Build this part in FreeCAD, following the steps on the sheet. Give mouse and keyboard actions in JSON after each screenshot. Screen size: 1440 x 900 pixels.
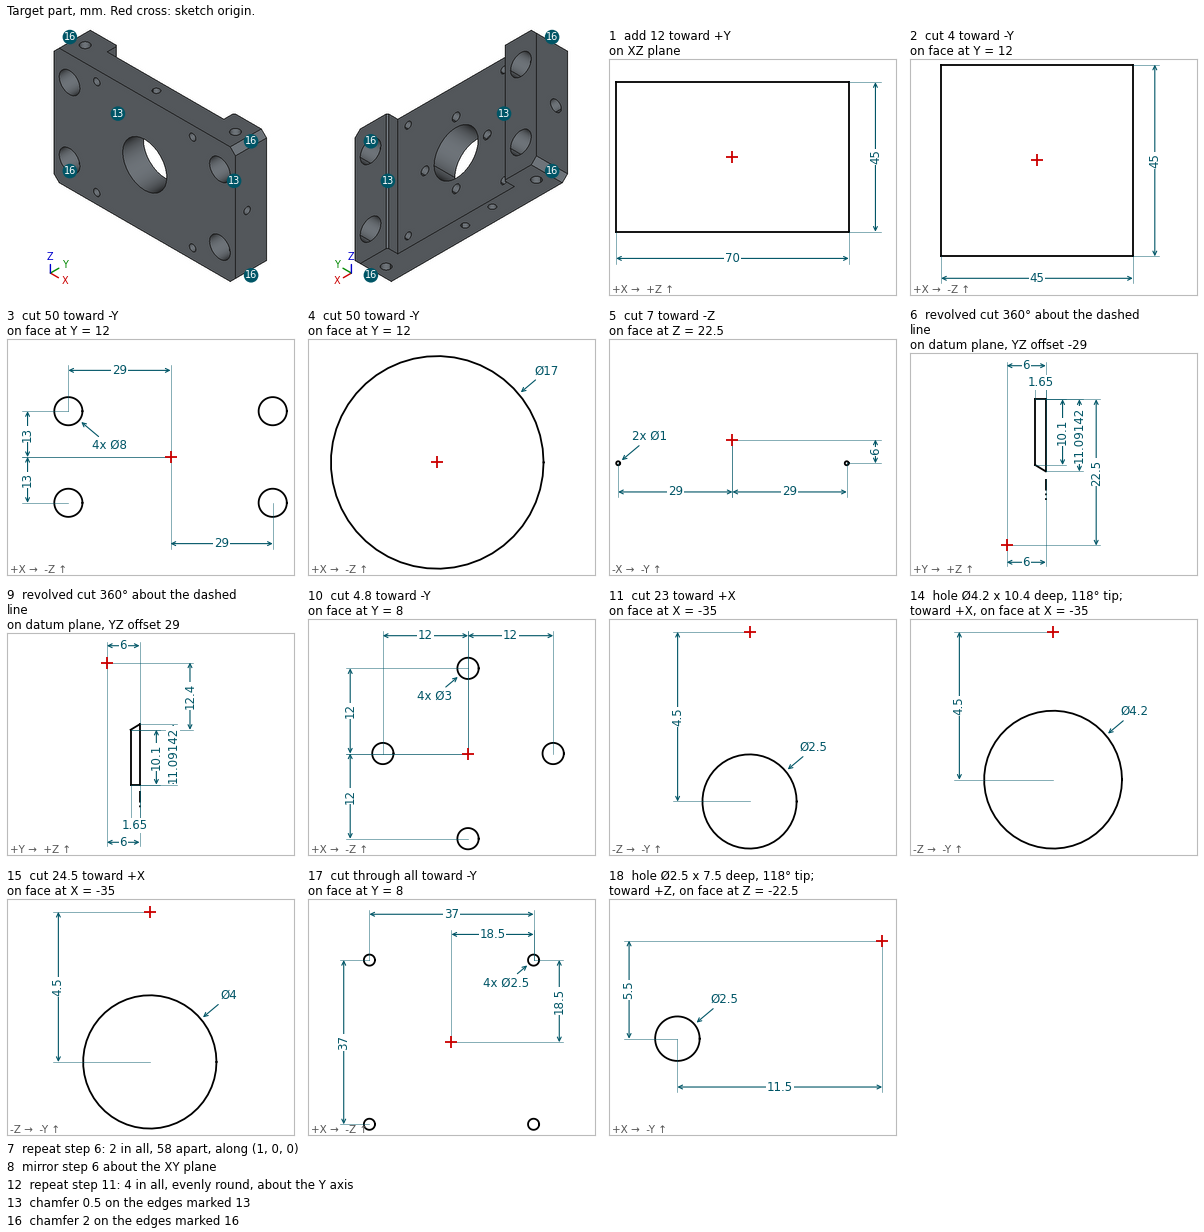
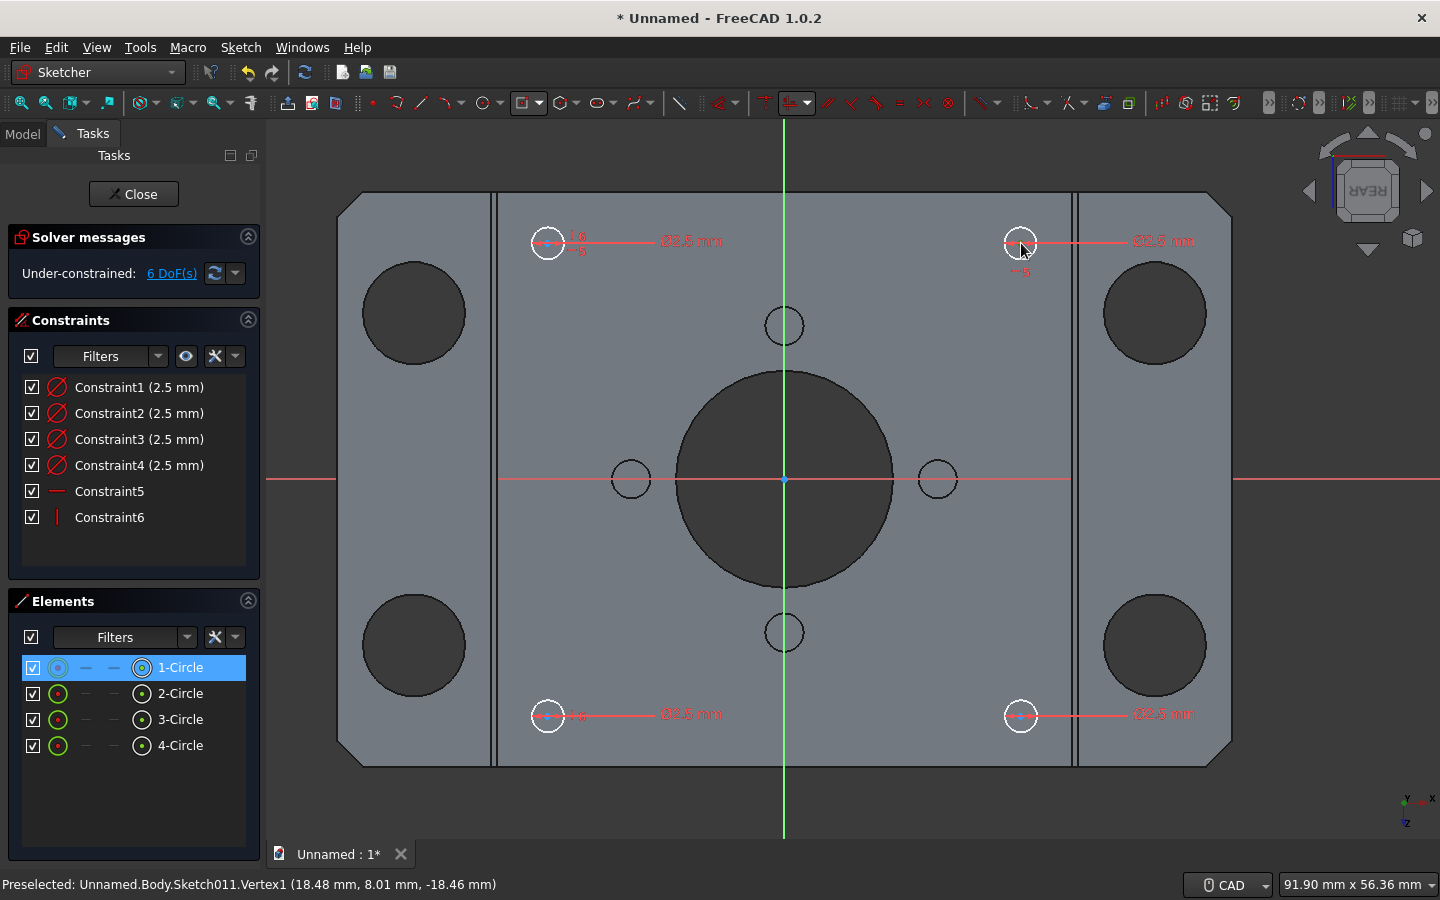
{"action": "left_click", "coordinate": [1021, 716]}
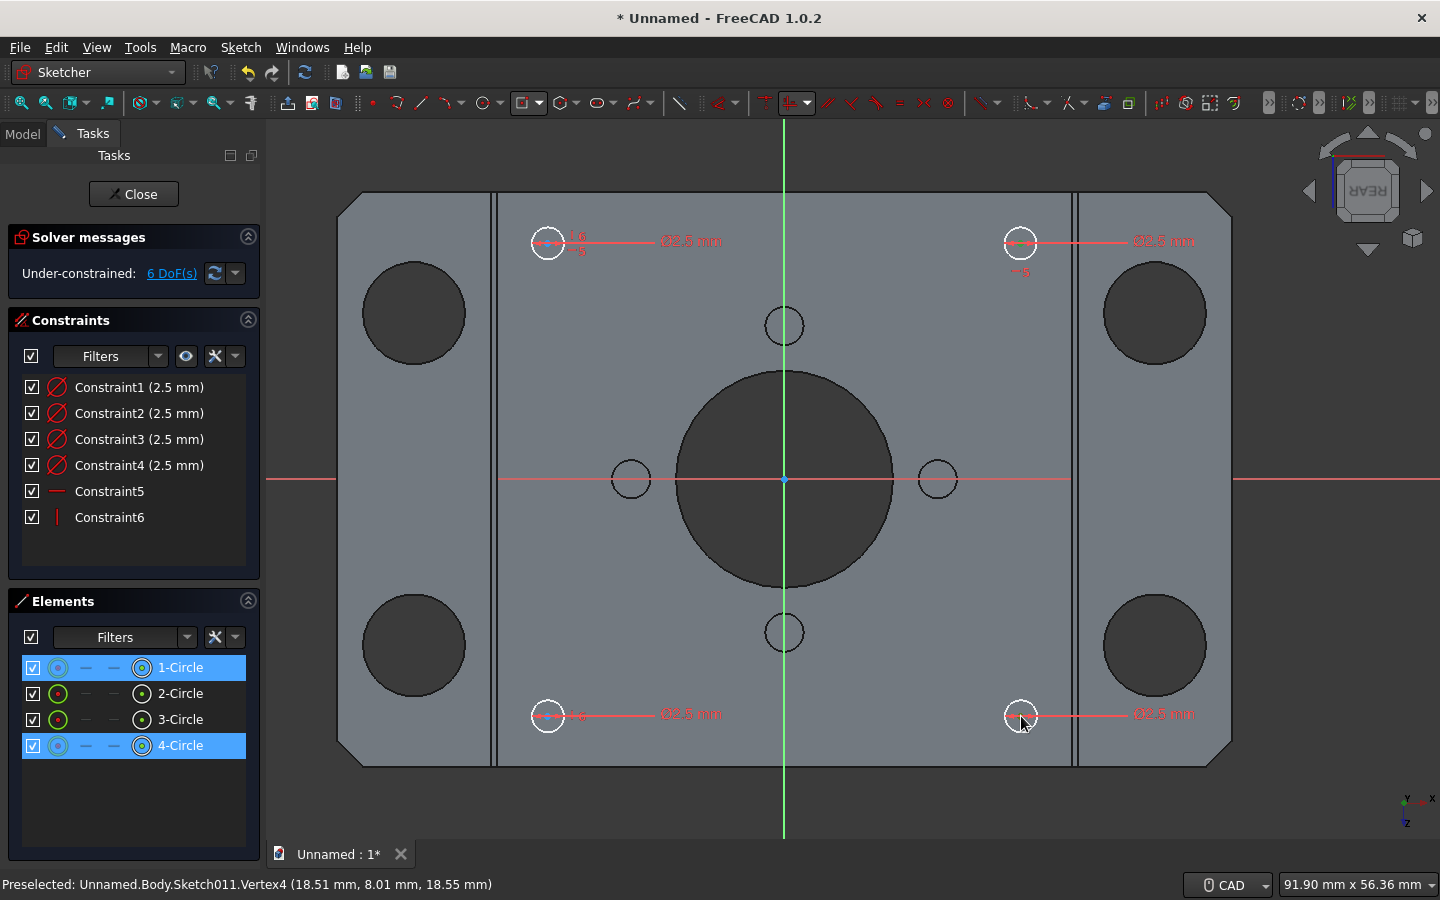
{"action": "left_click", "coordinate": [810, 104]}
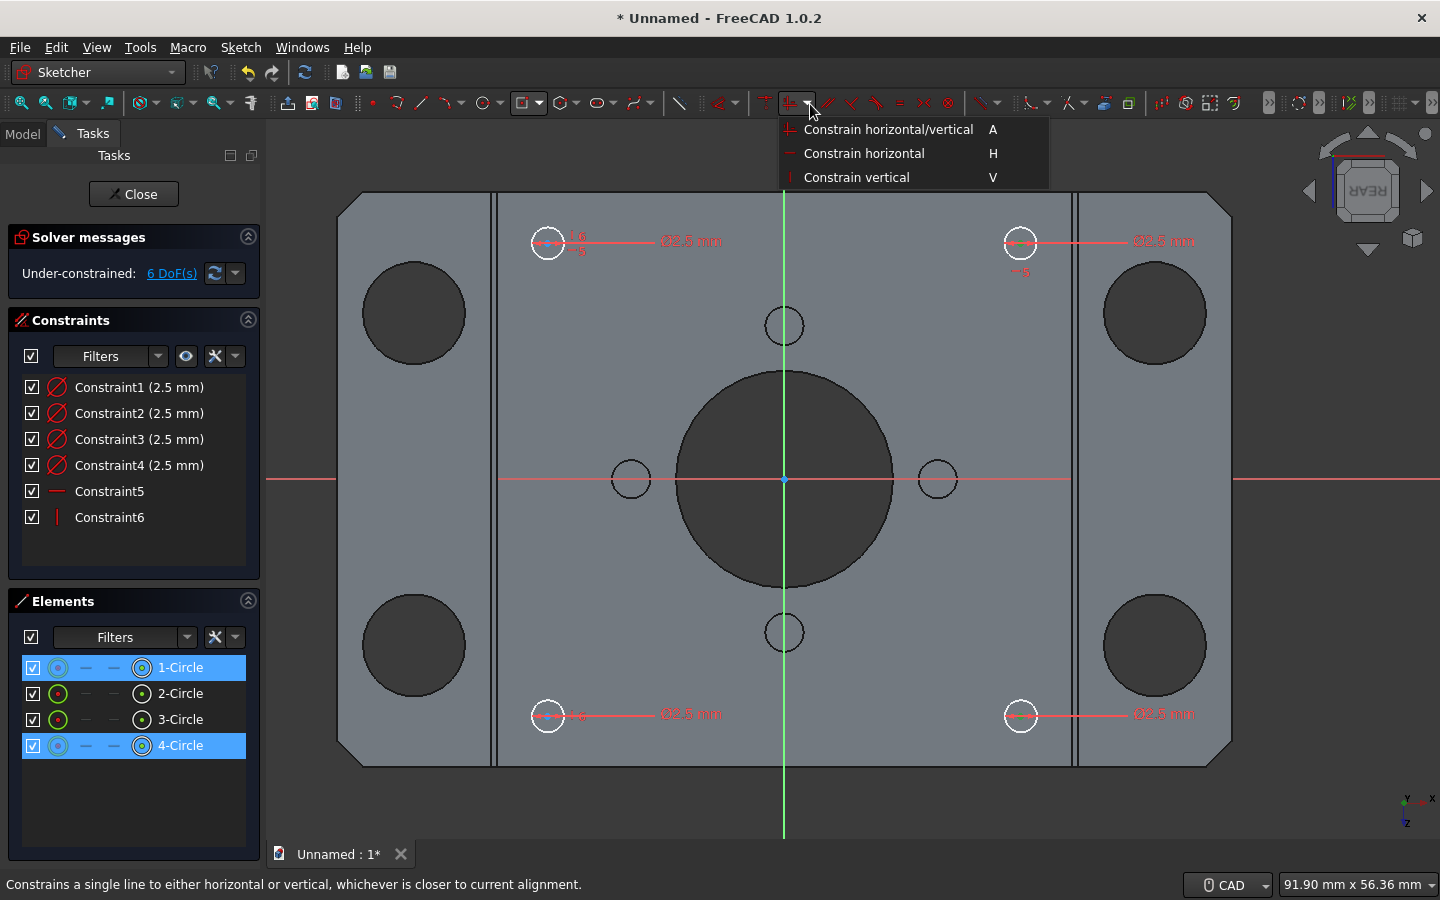
{"action": "left_click", "coordinate": [914, 177]}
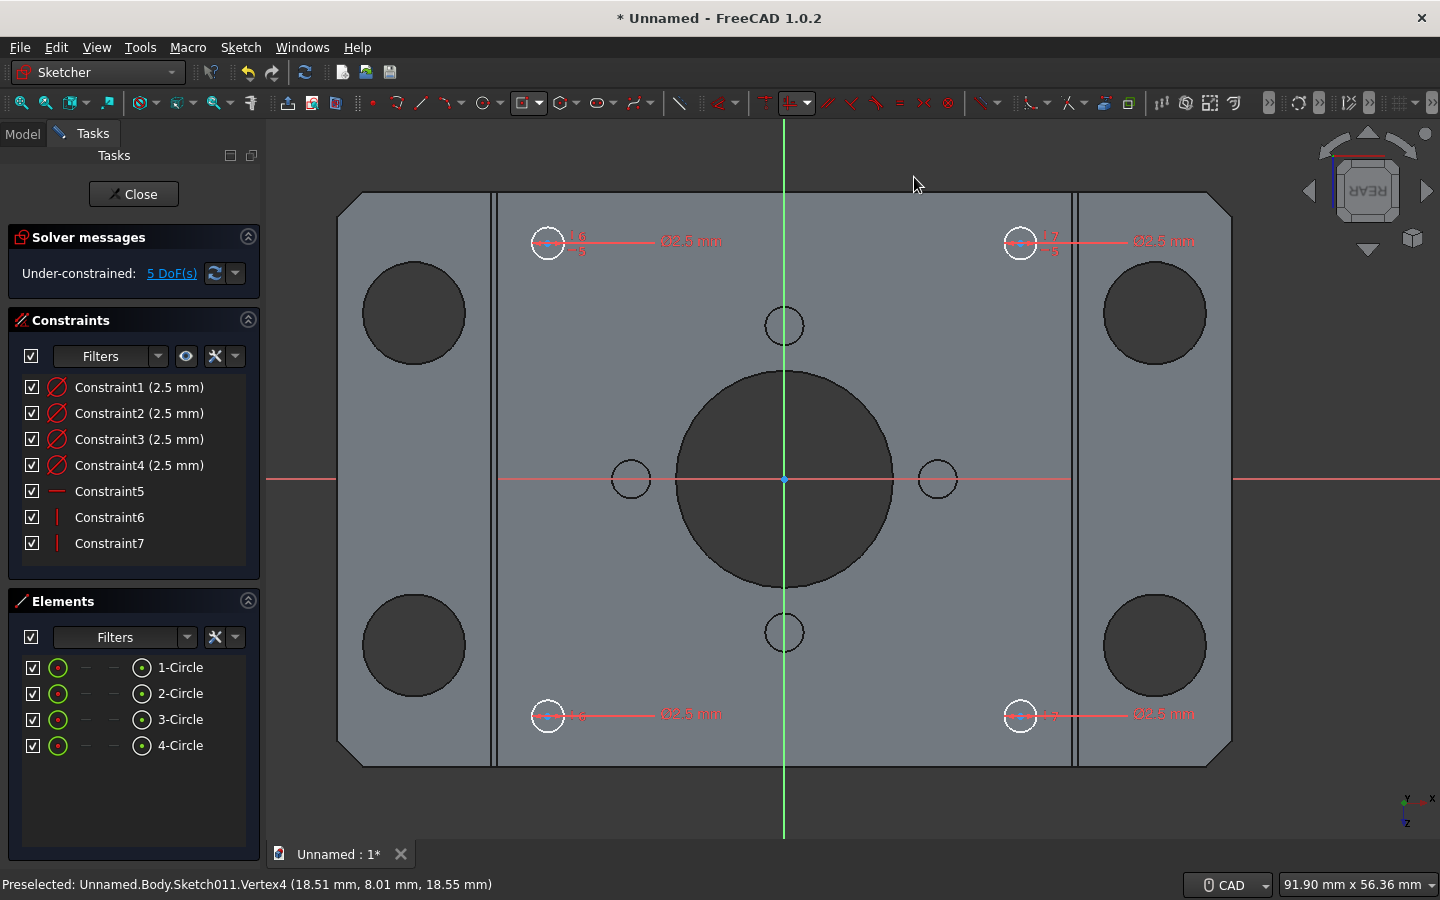
{"action": "left_click", "coordinate": [548, 716]}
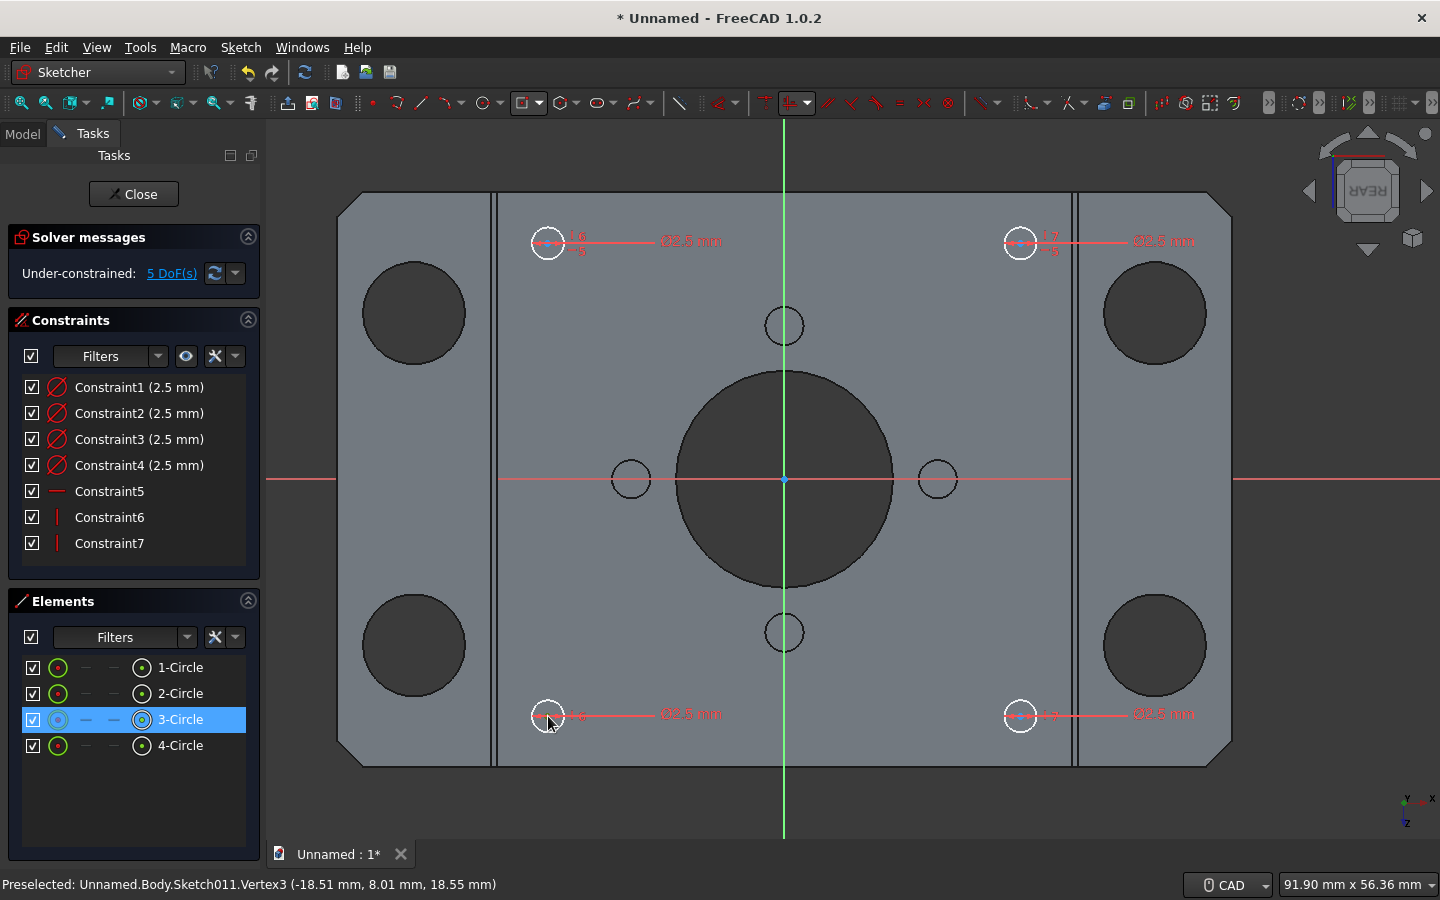
{"action": "left_click", "coordinate": [1021, 716]}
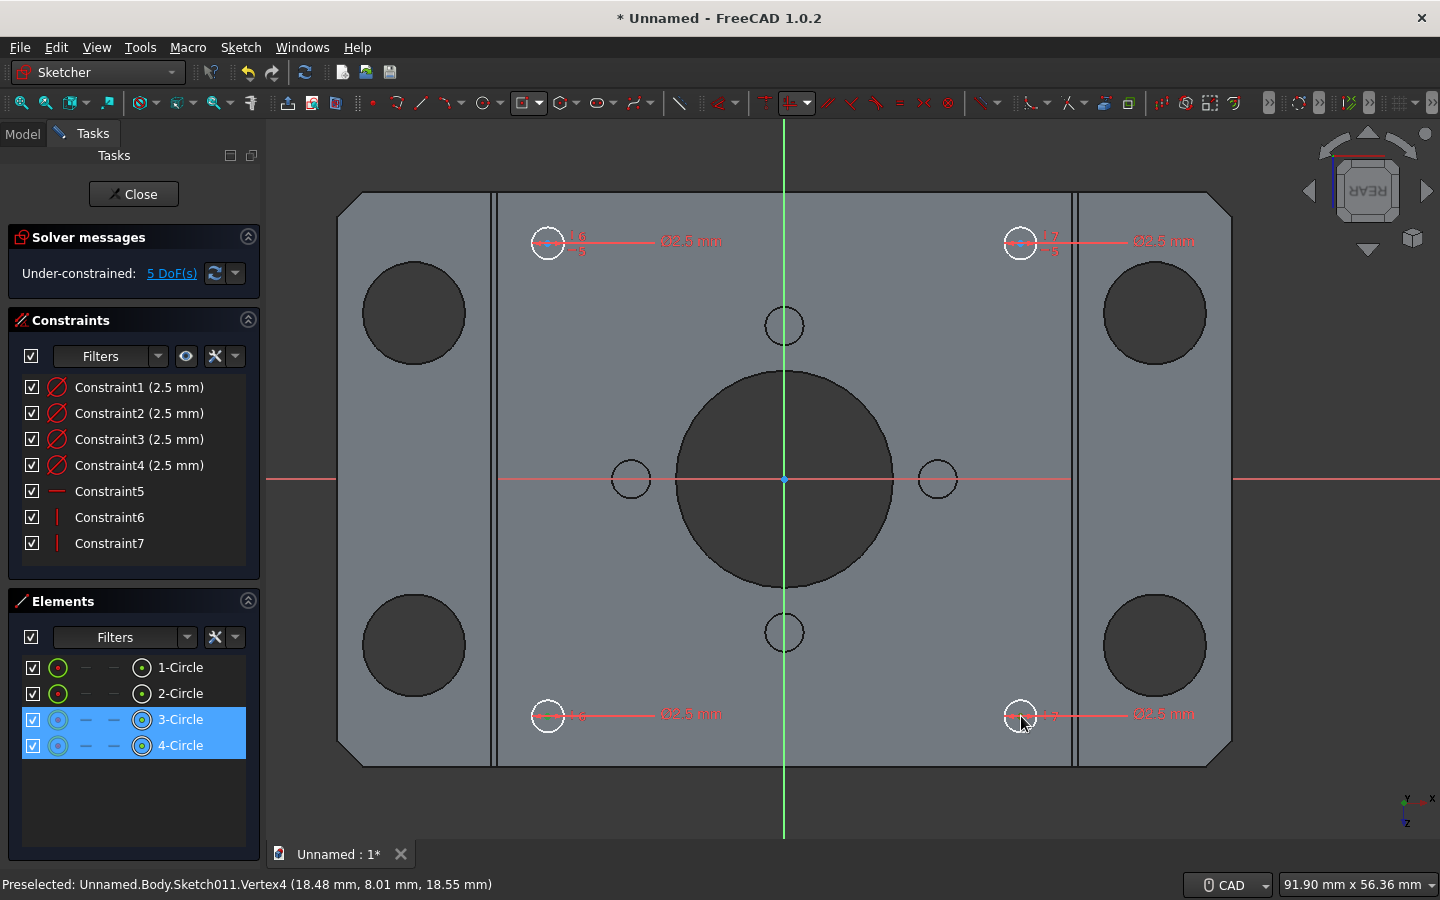
{"action": "key", "text": "h"}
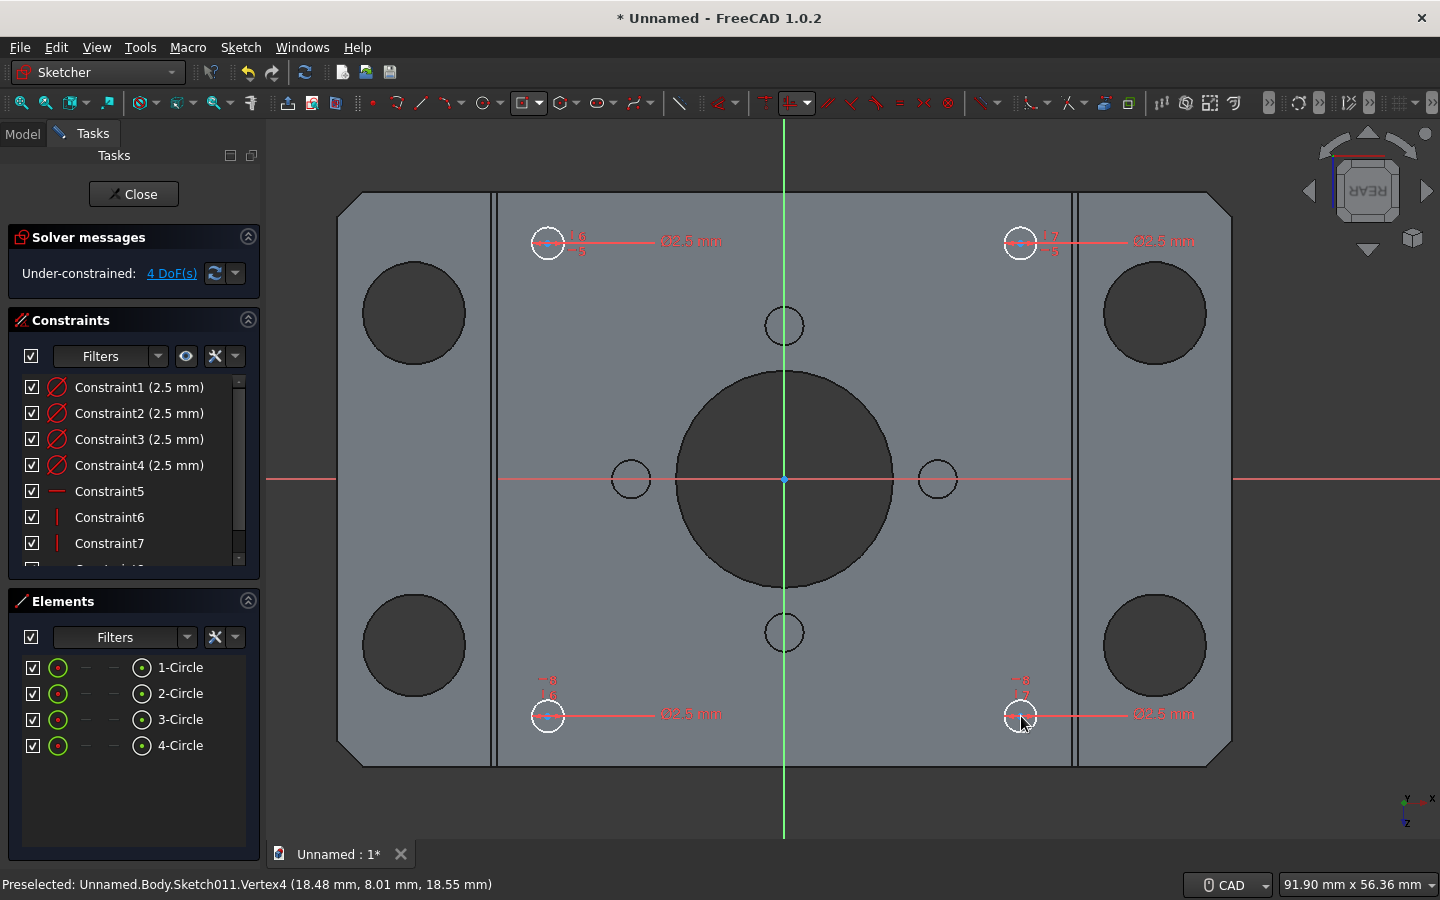
{"action": "left_click", "coordinate": [718, 104]}